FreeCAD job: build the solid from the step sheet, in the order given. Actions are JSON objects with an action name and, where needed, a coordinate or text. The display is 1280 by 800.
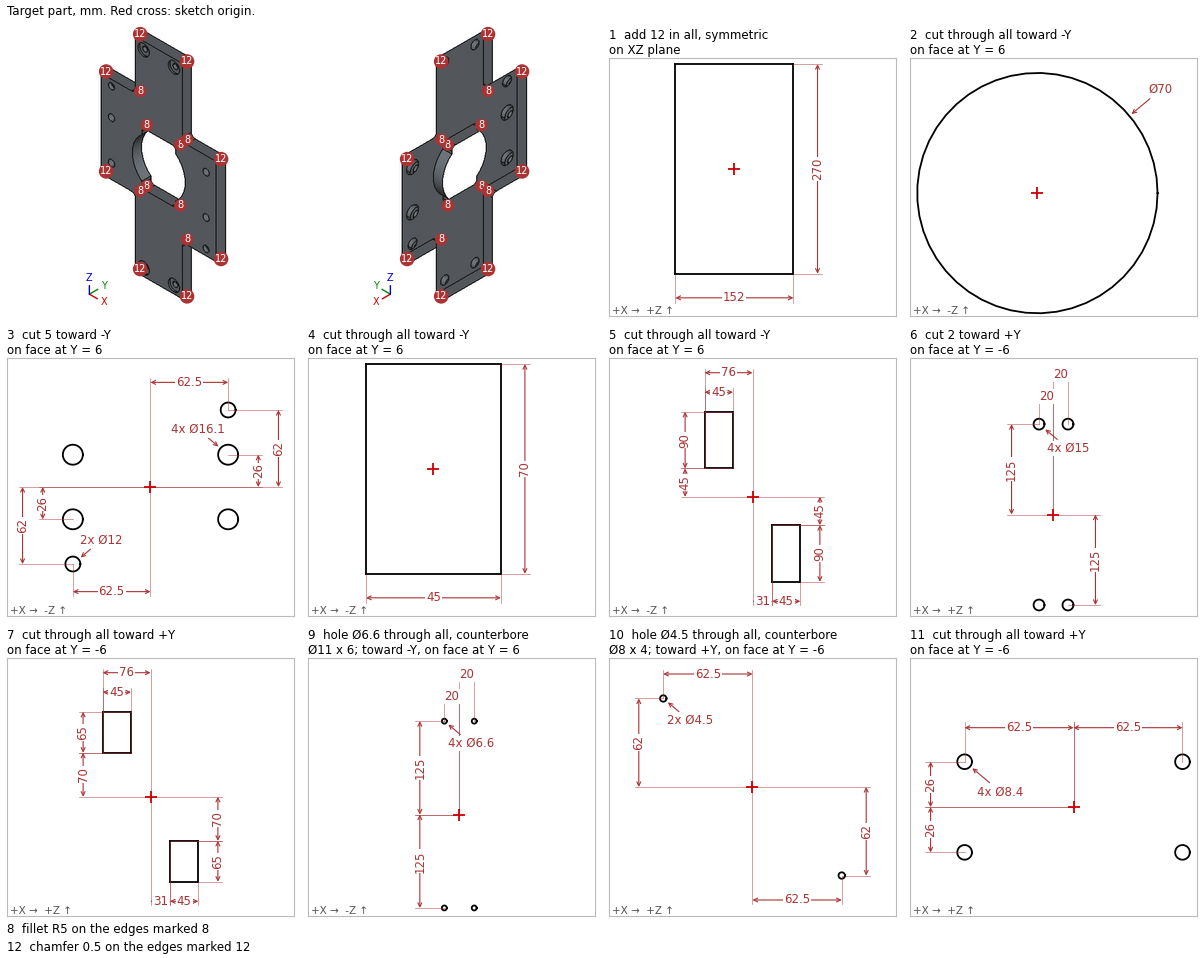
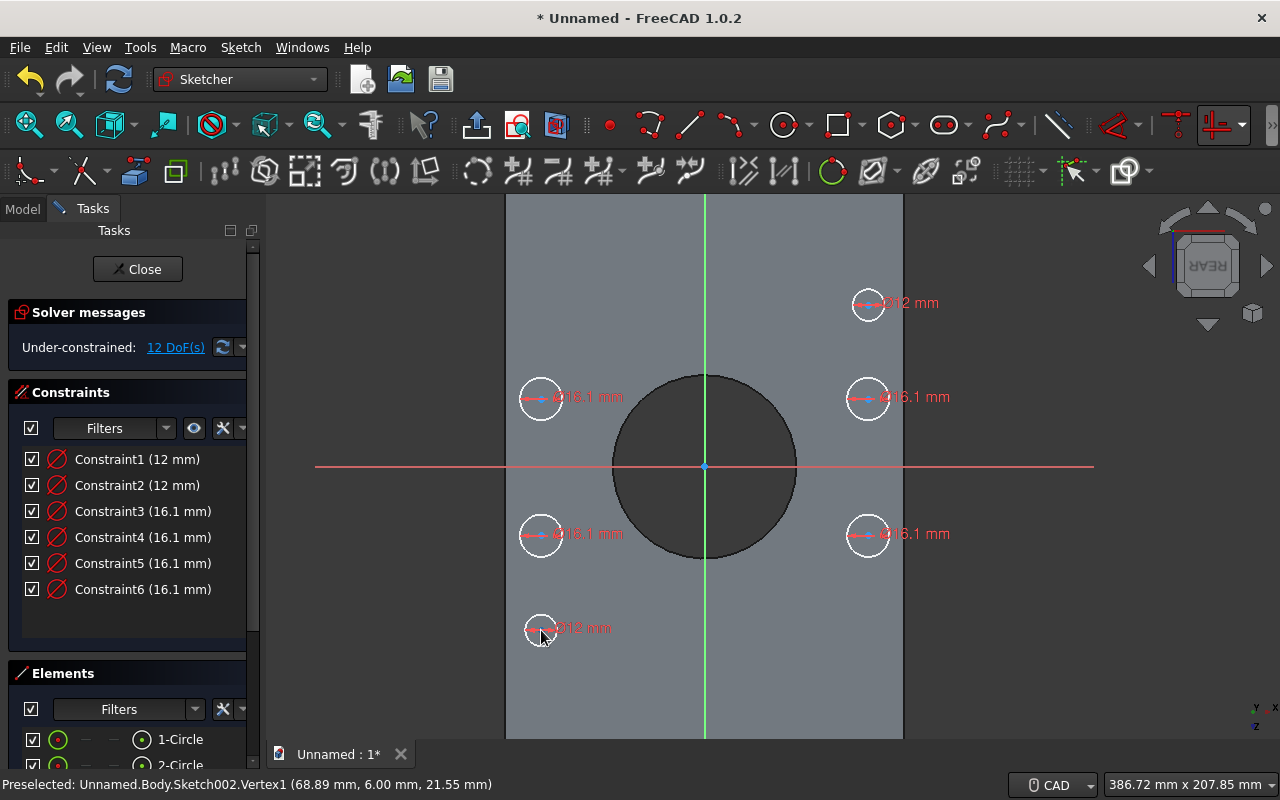
{"action": "left_click", "coordinate": [869, 305]}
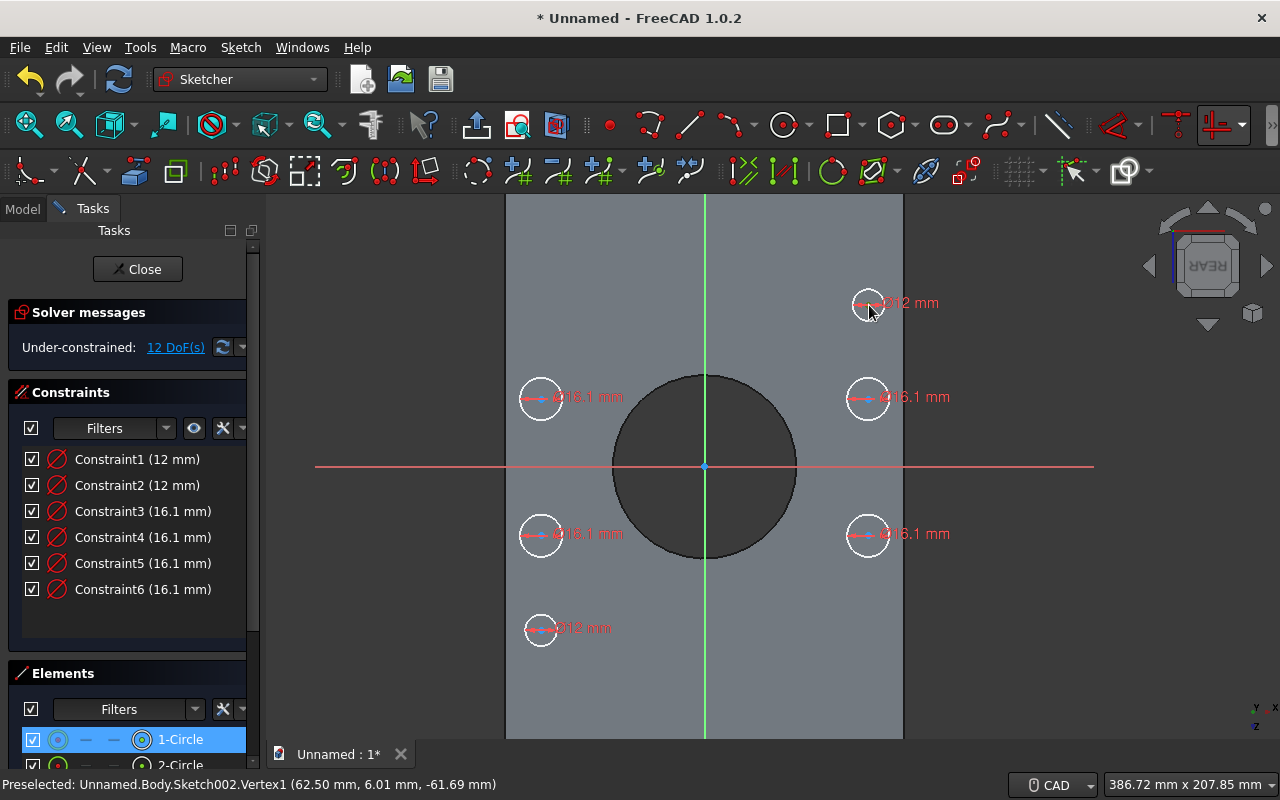
{"action": "left_click", "coordinate": [868, 399]}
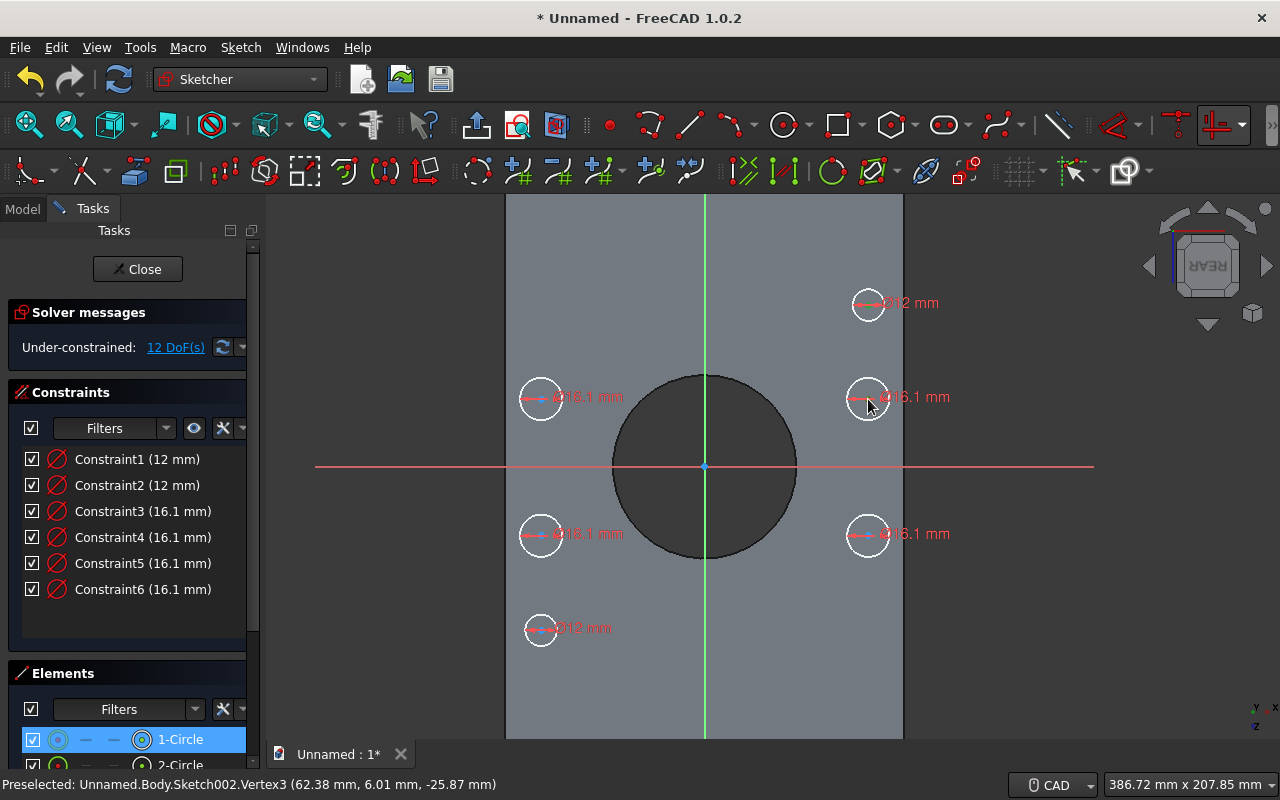
{"action": "left_click", "coordinate": [1244, 126]}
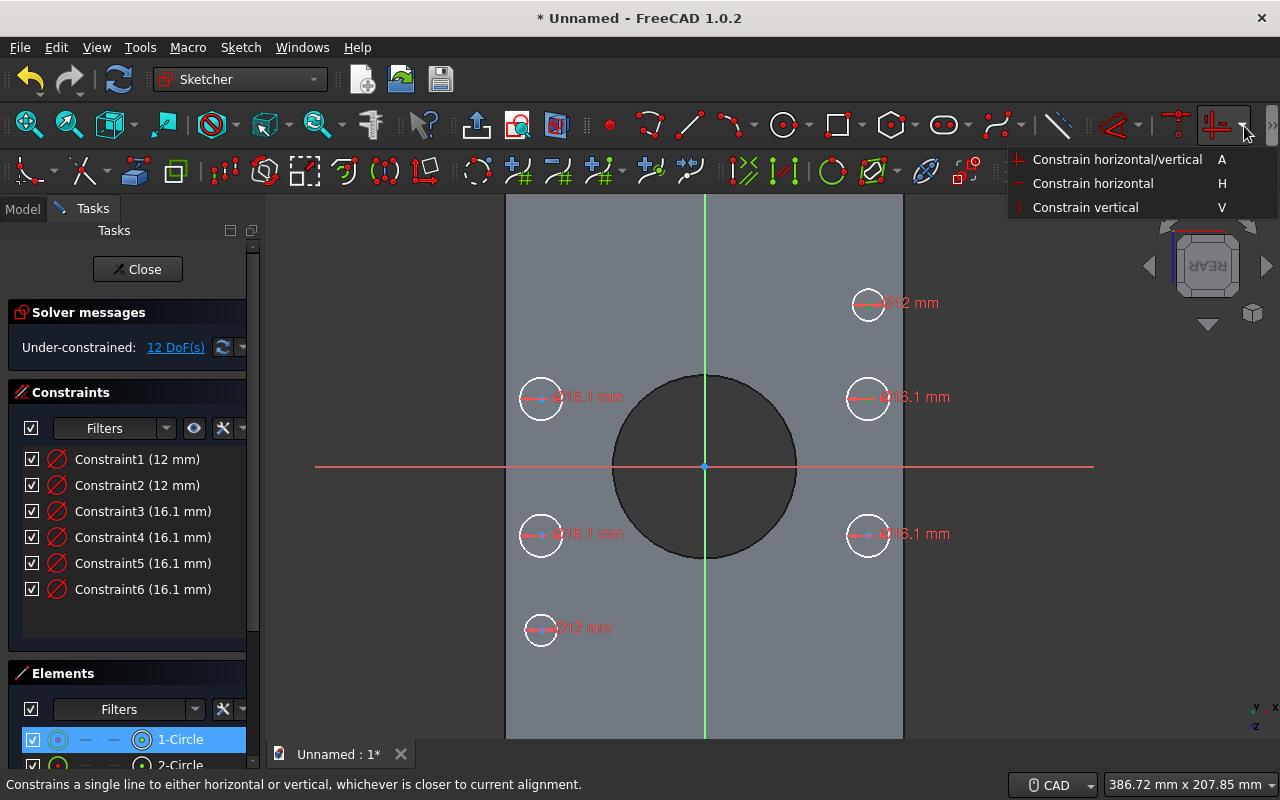
{"action": "left_click", "coordinate": [1143, 207]}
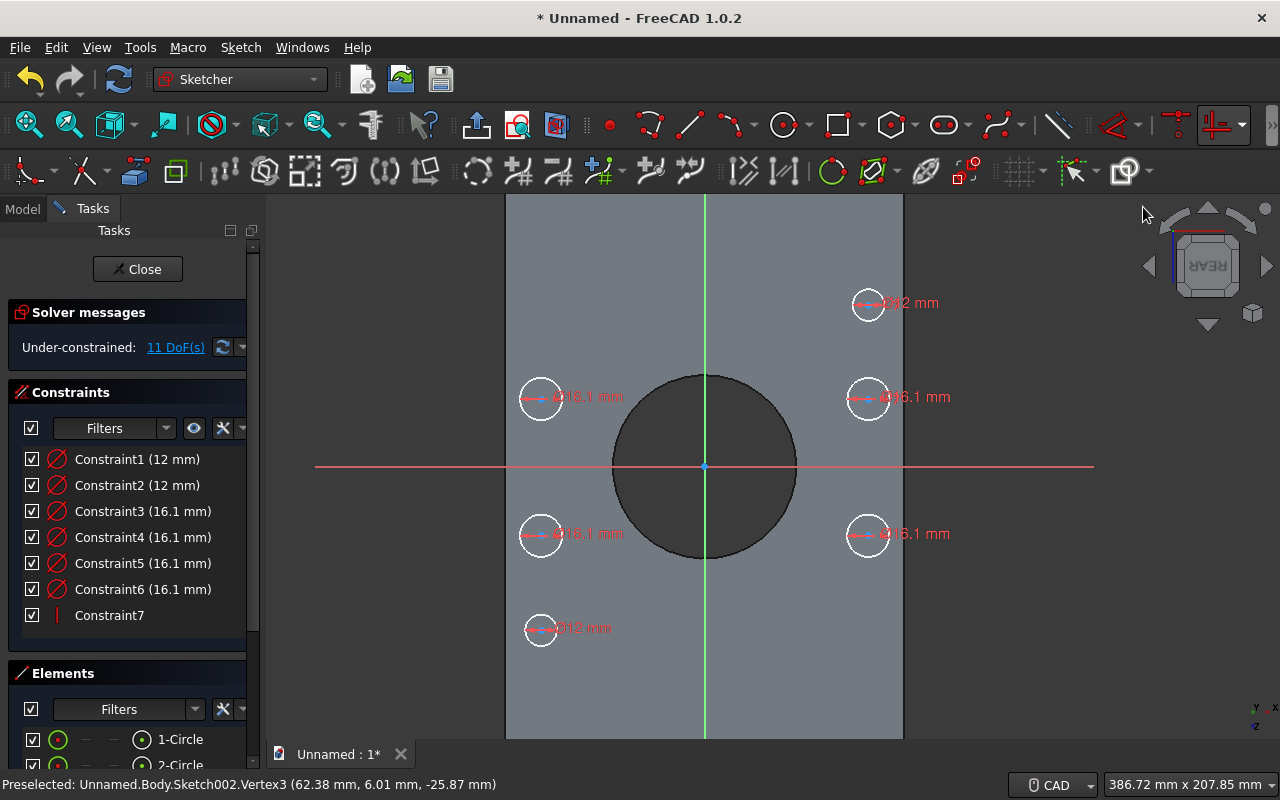
{"action": "left_click", "coordinate": [541, 630]}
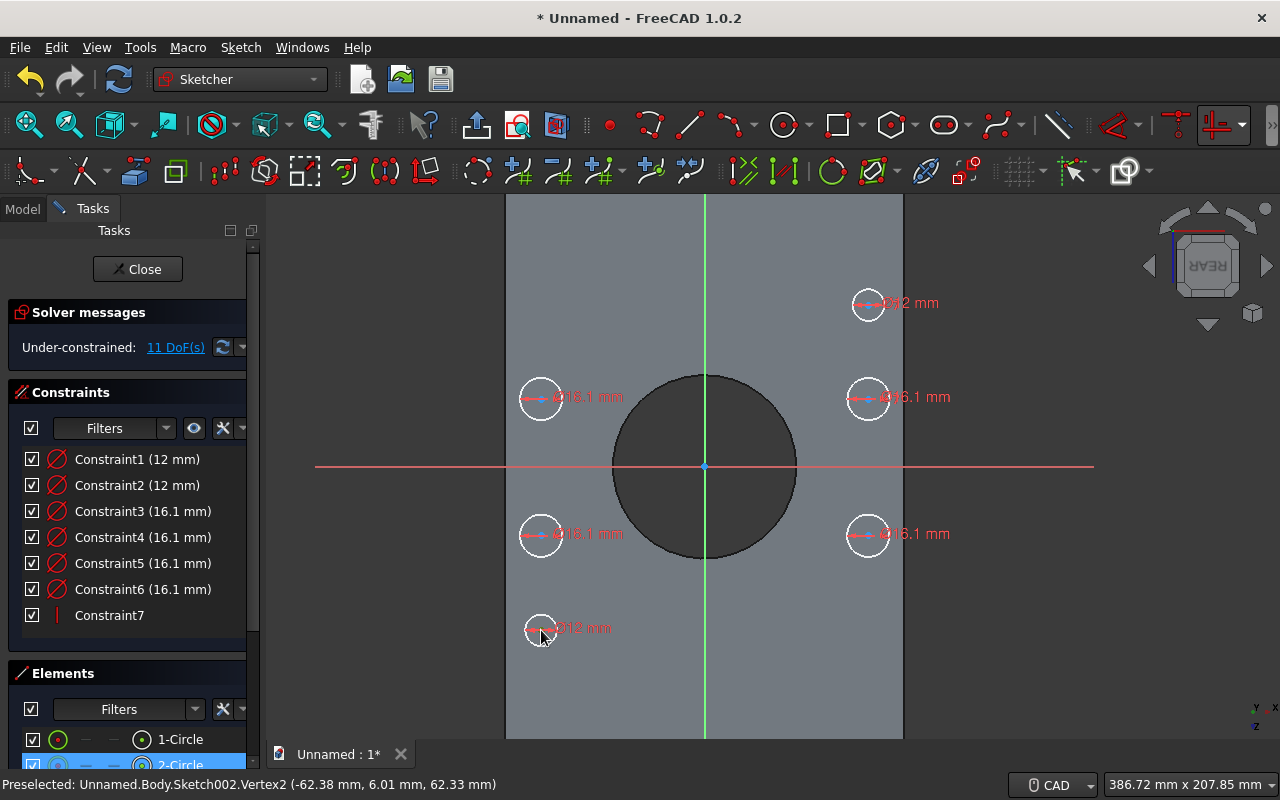
{"action": "left_click", "coordinate": [541, 399]}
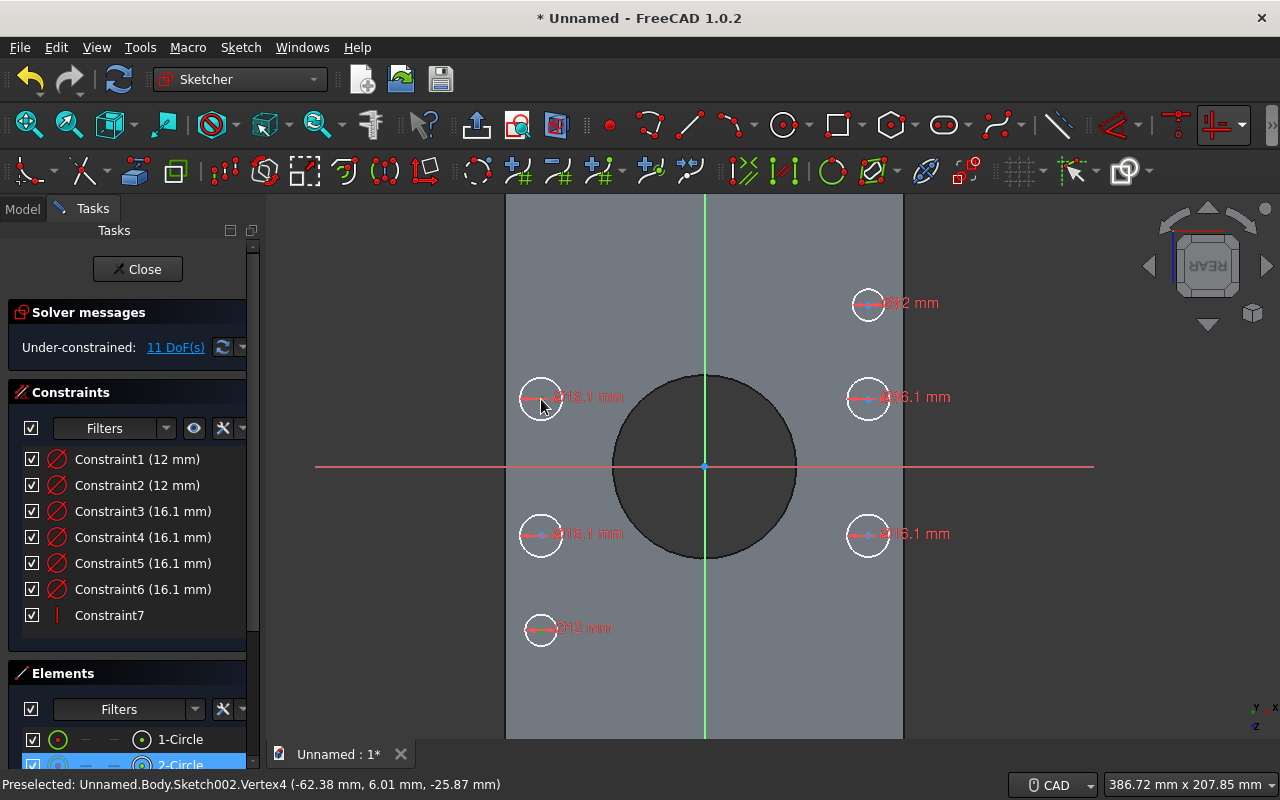
{"action": "key", "text": "v"}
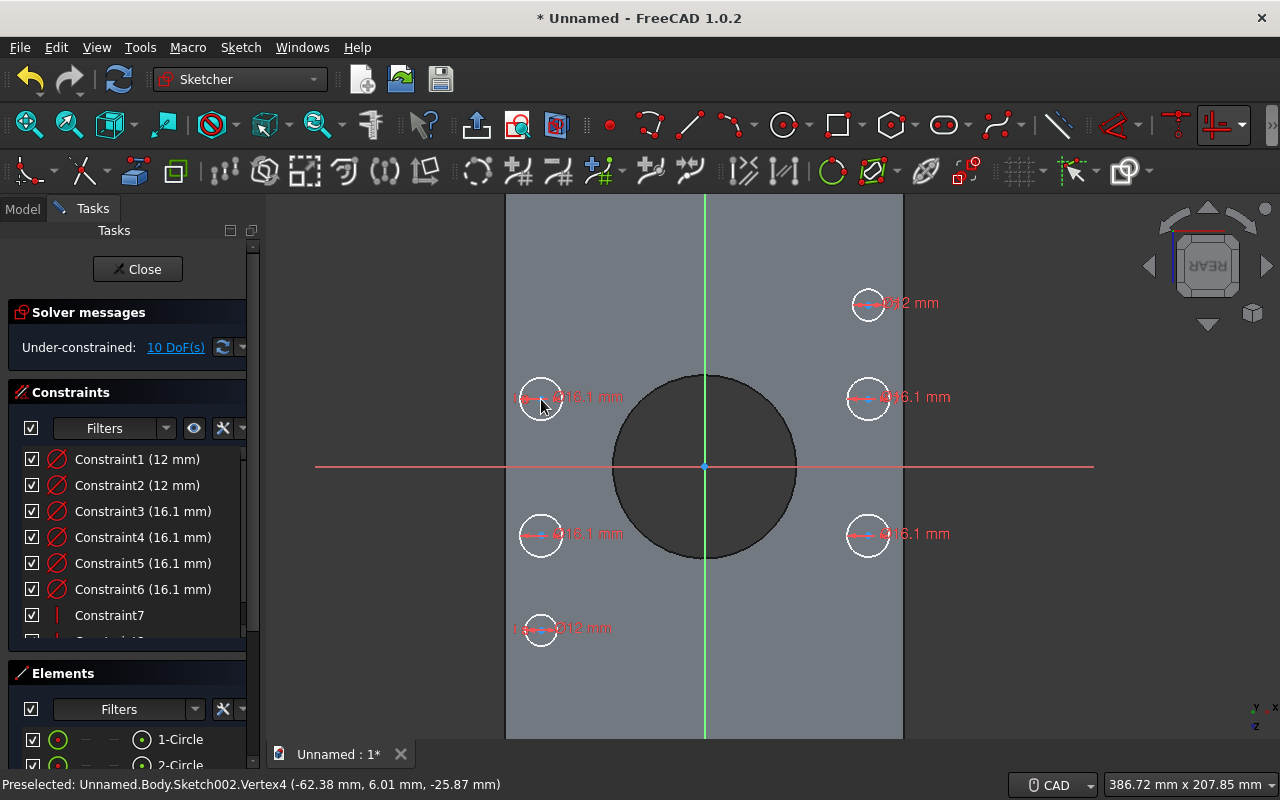
{"action": "left_click", "coordinate": [869, 399]}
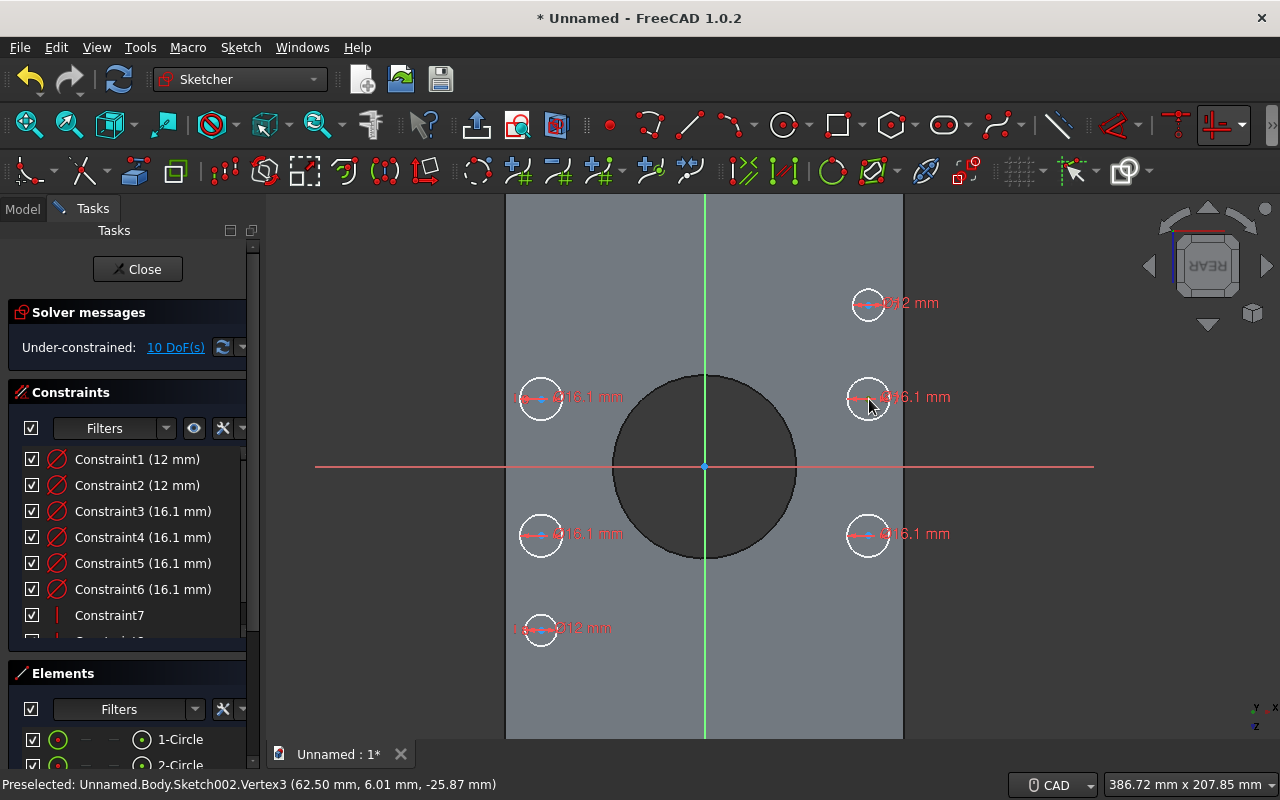
{"action": "left_click", "coordinate": [541, 399]}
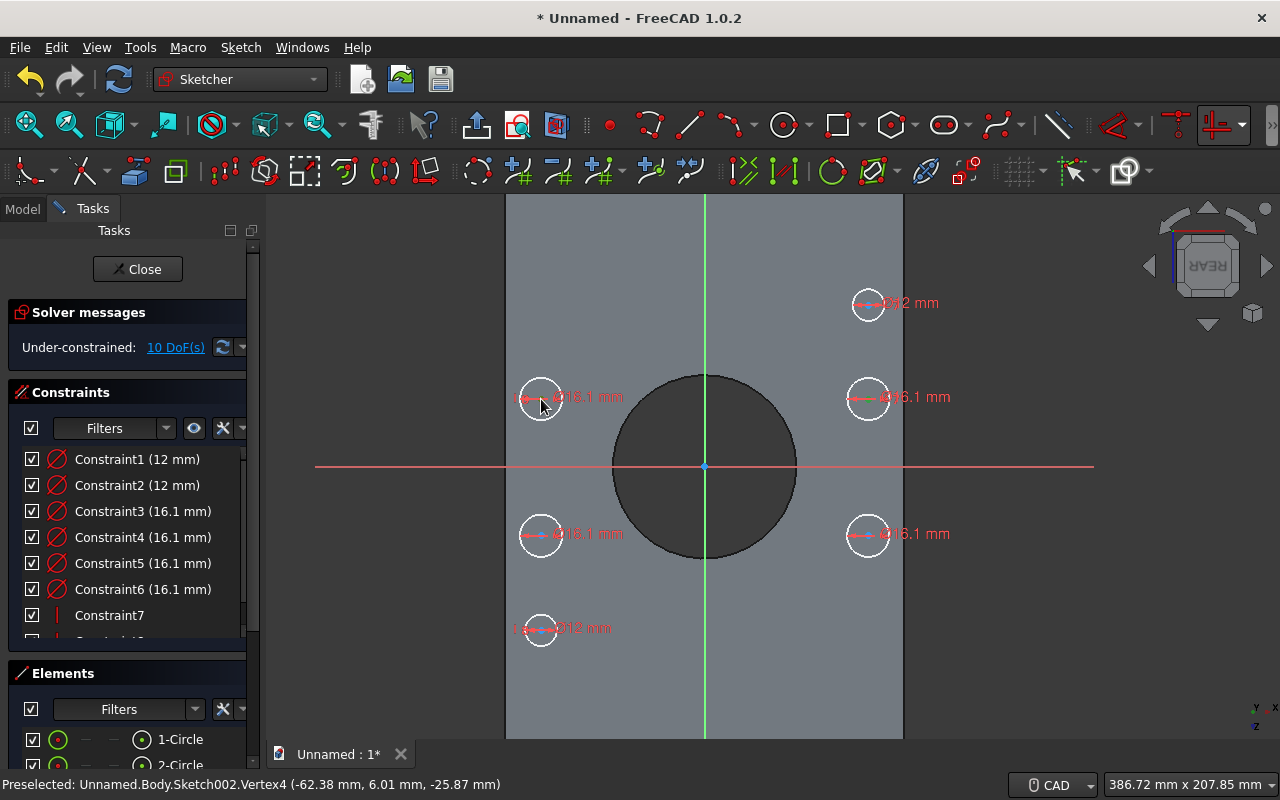
{"action": "key", "text": "h"}